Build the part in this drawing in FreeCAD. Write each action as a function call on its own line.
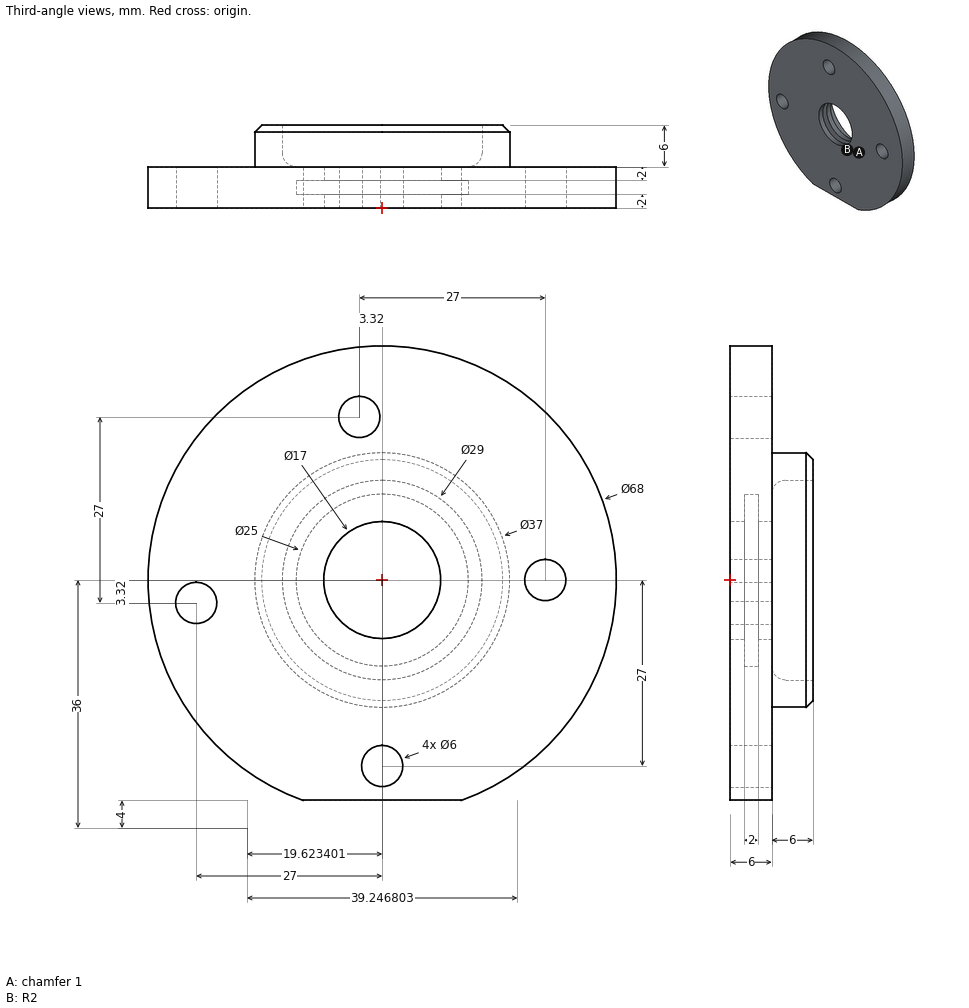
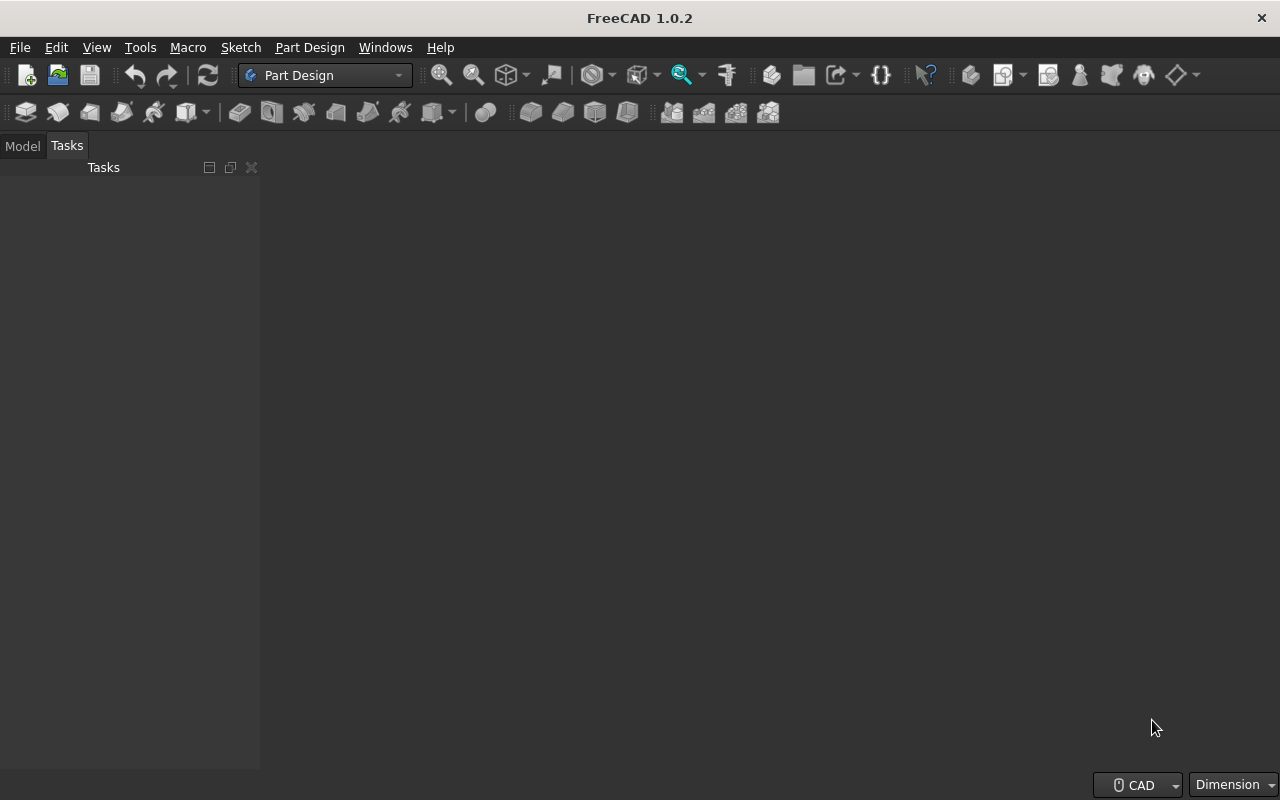
click(26, 76)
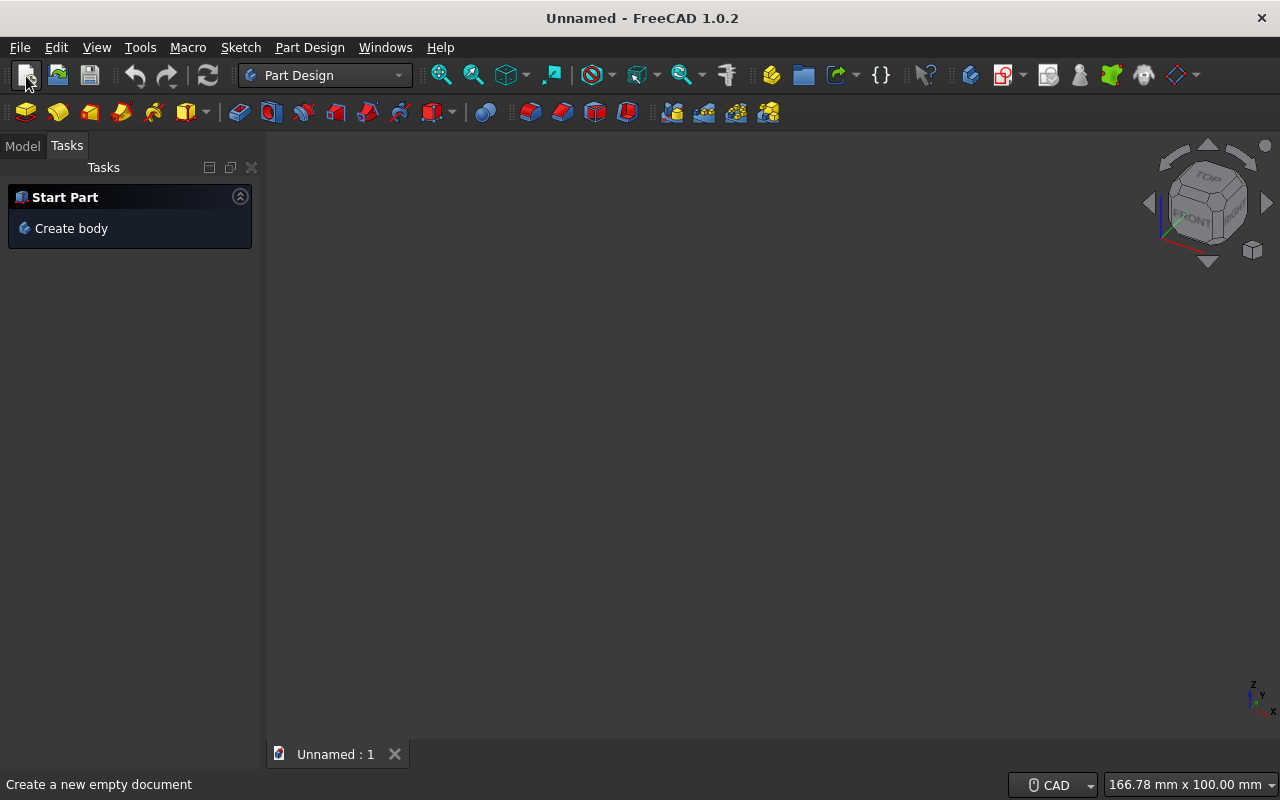
click(1004, 76)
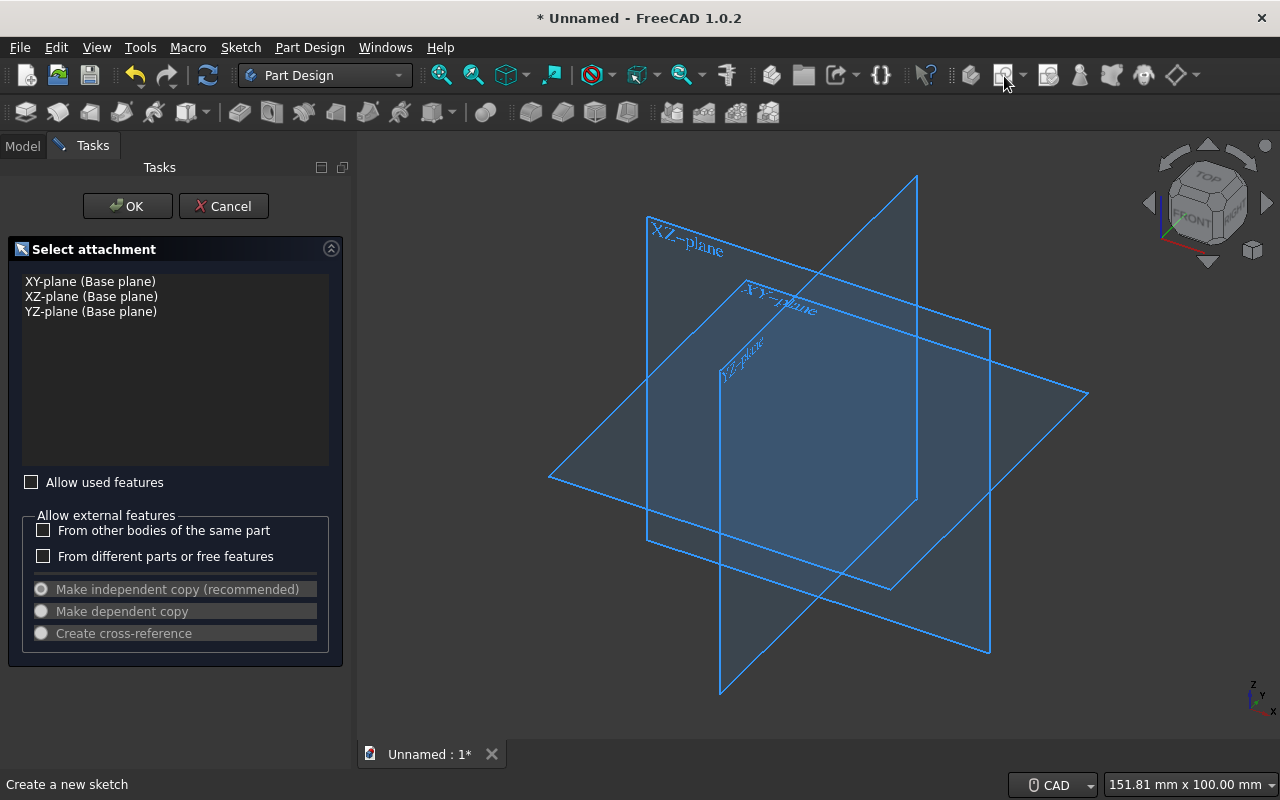
click(82, 296)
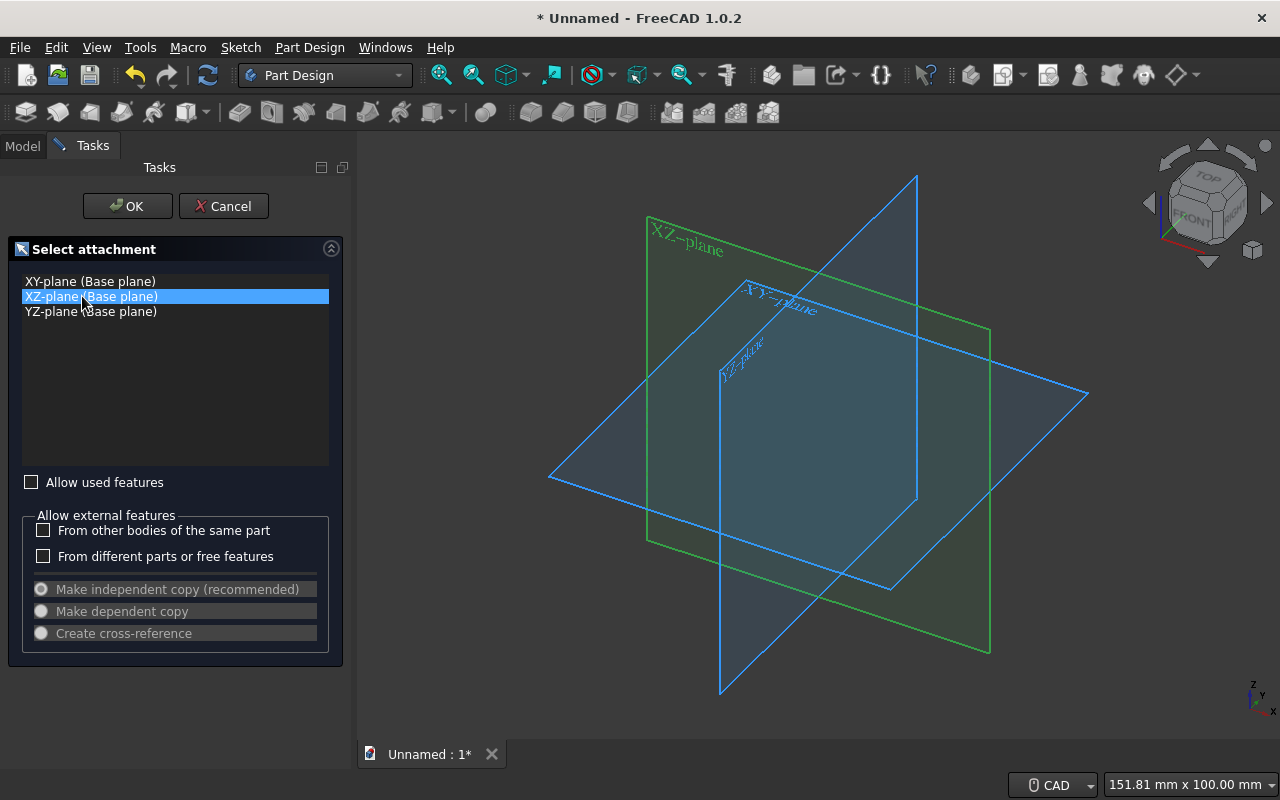
click(128, 206)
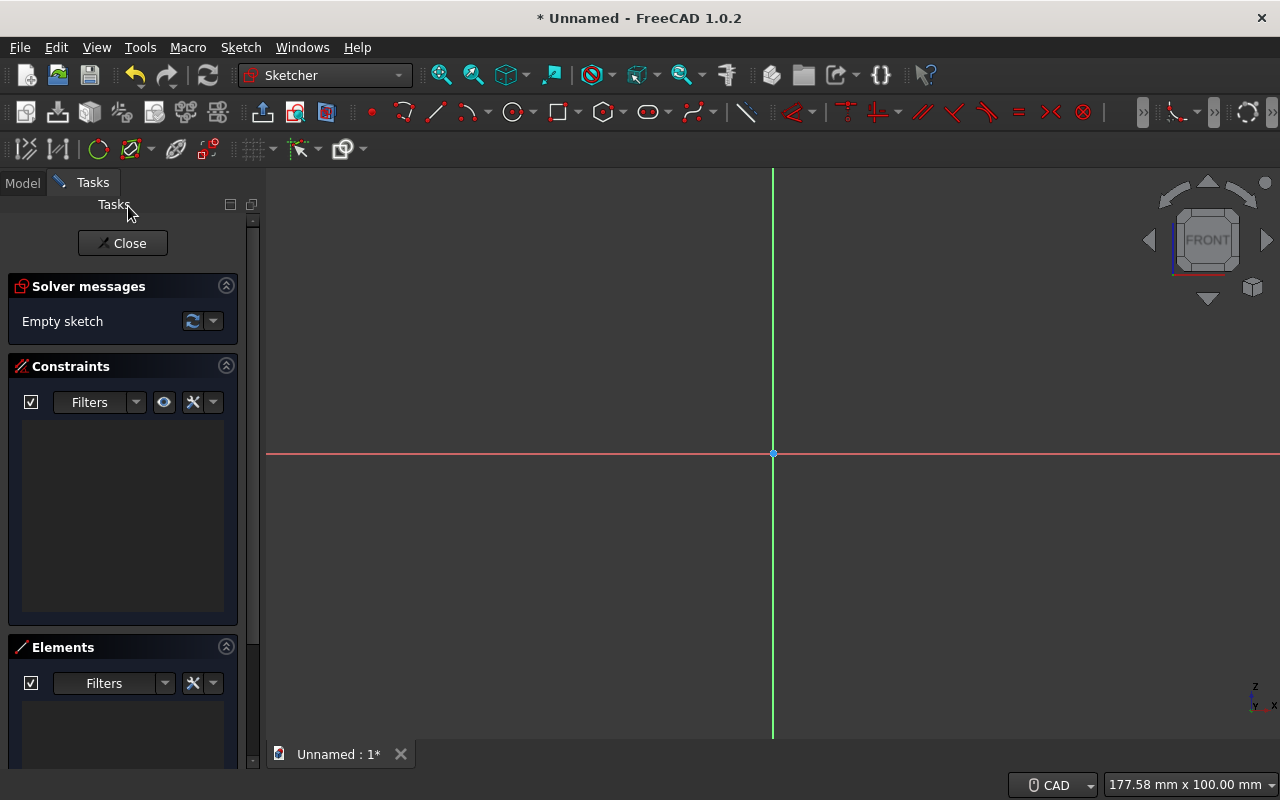
click(514, 112)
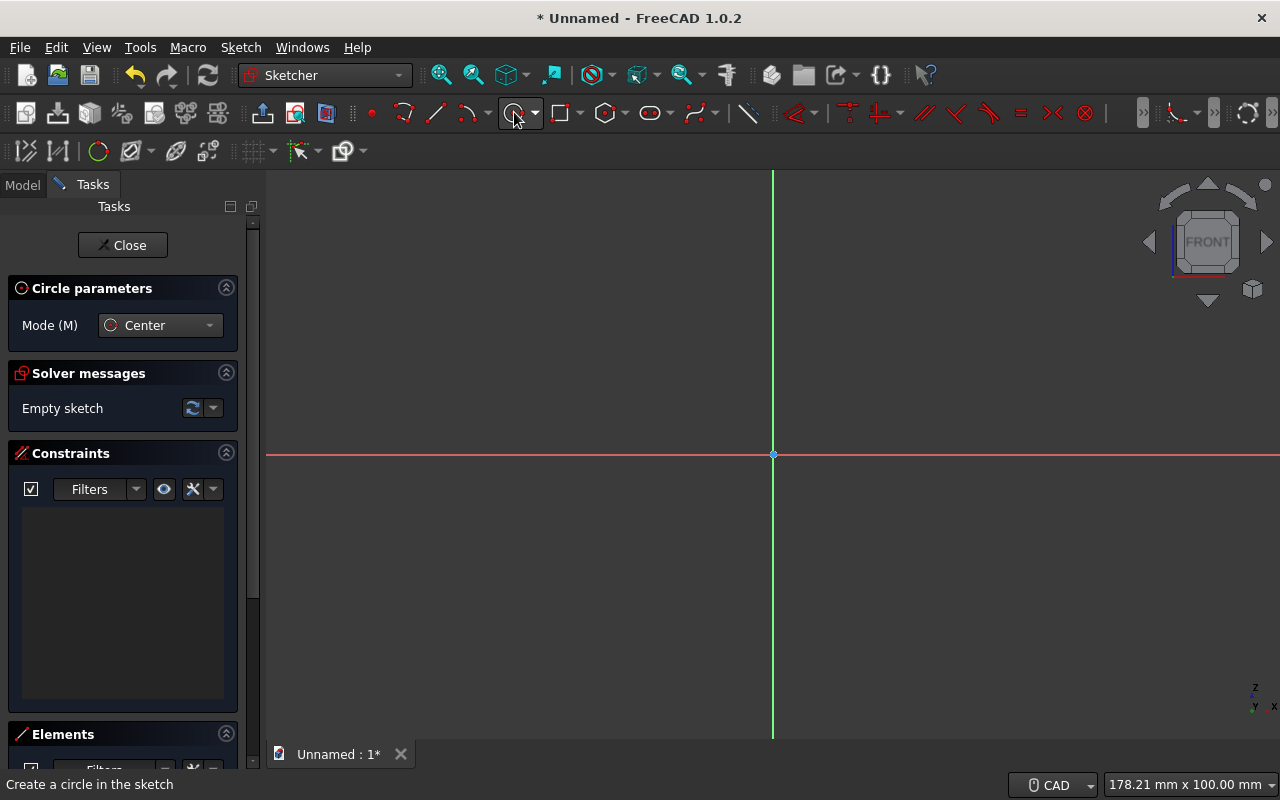
click(773, 454)
click(910, 318)
key(Escape)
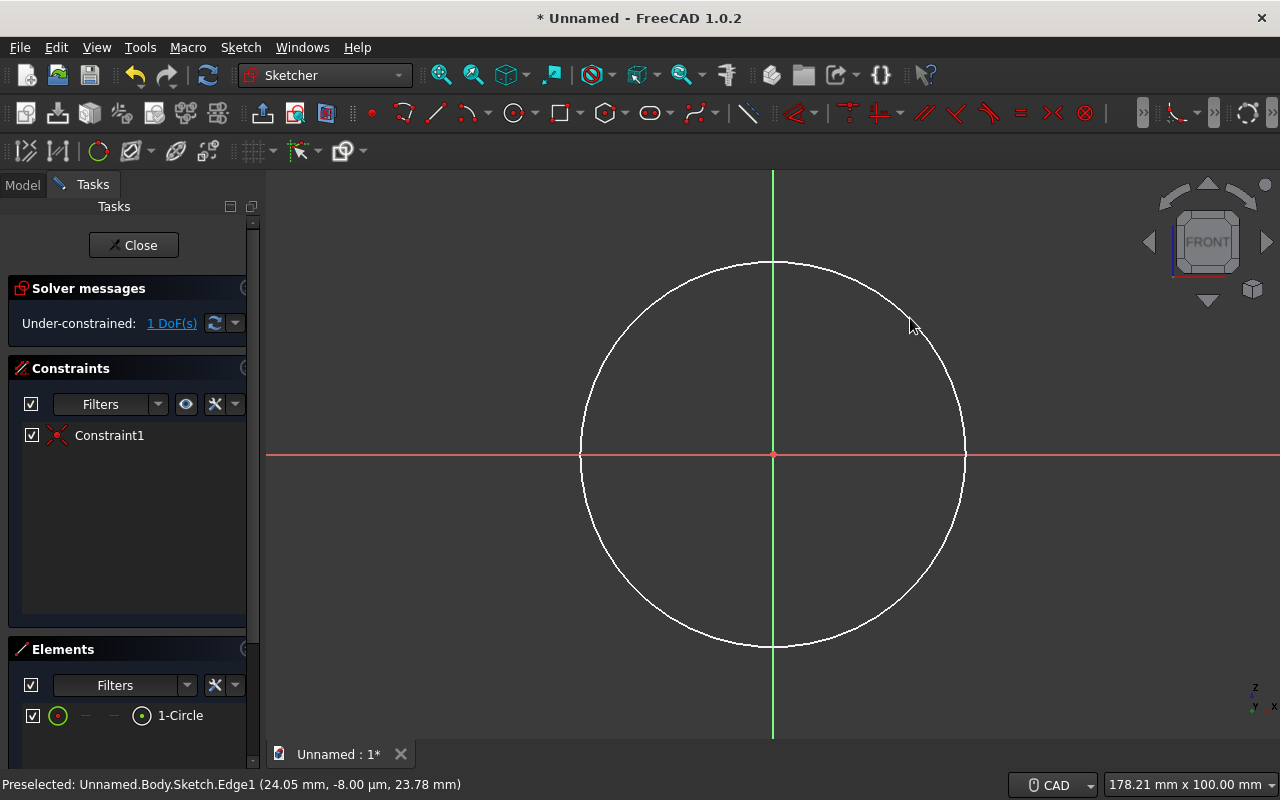
click(794, 114)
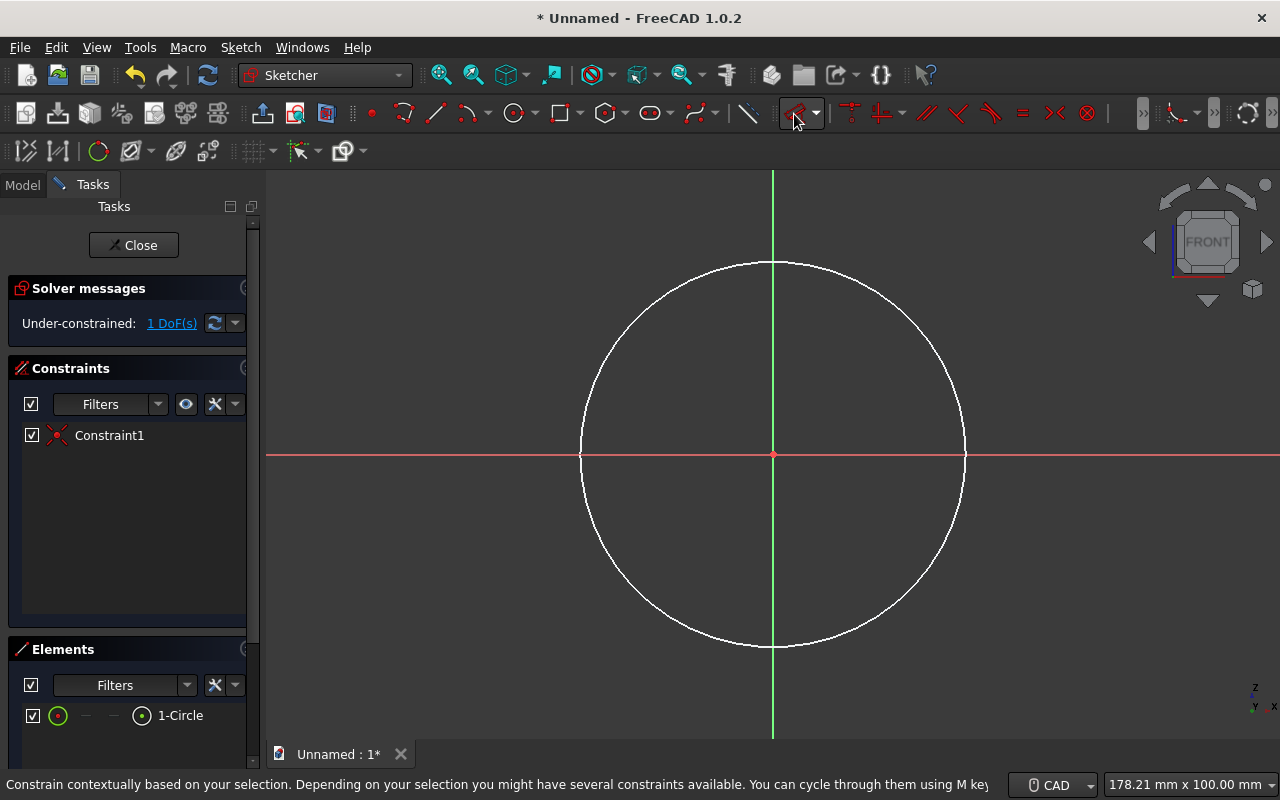
click(909, 318)
click(932, 295)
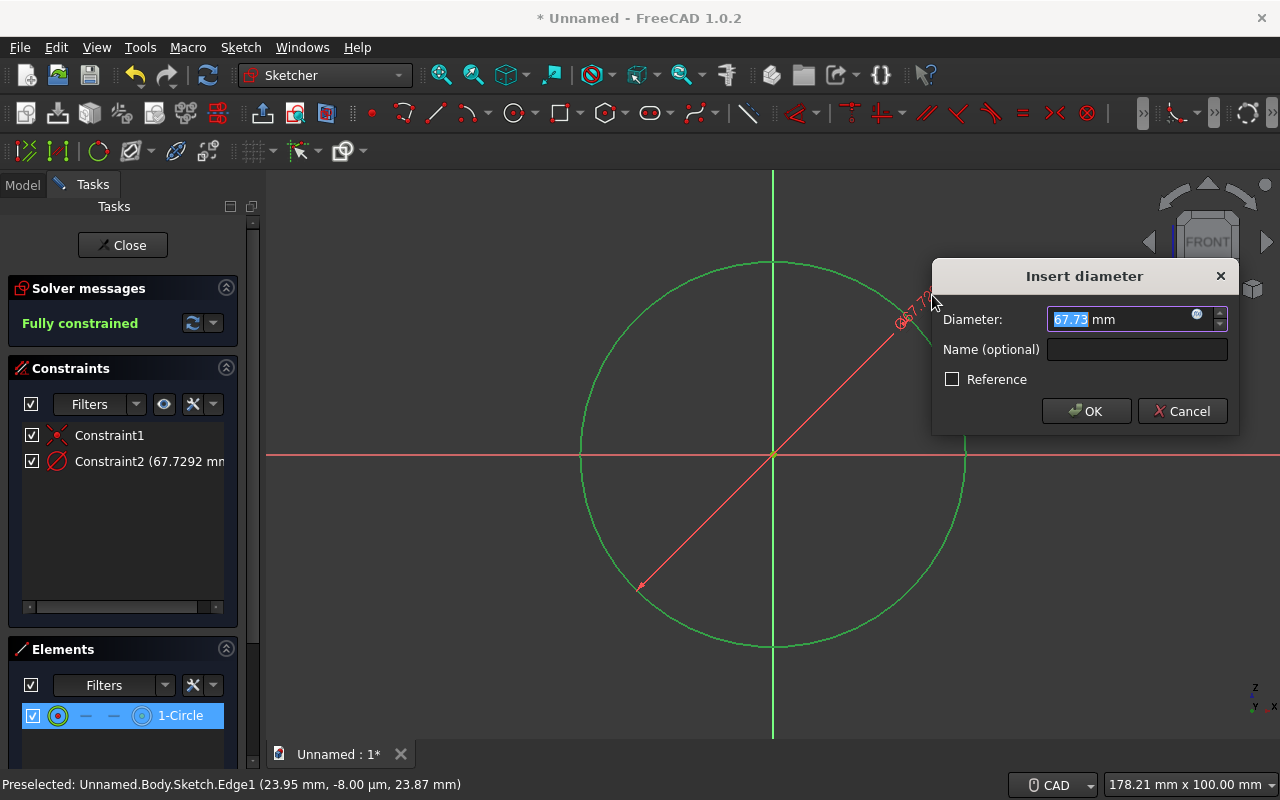
text(68)
key(Return)
key(Escape)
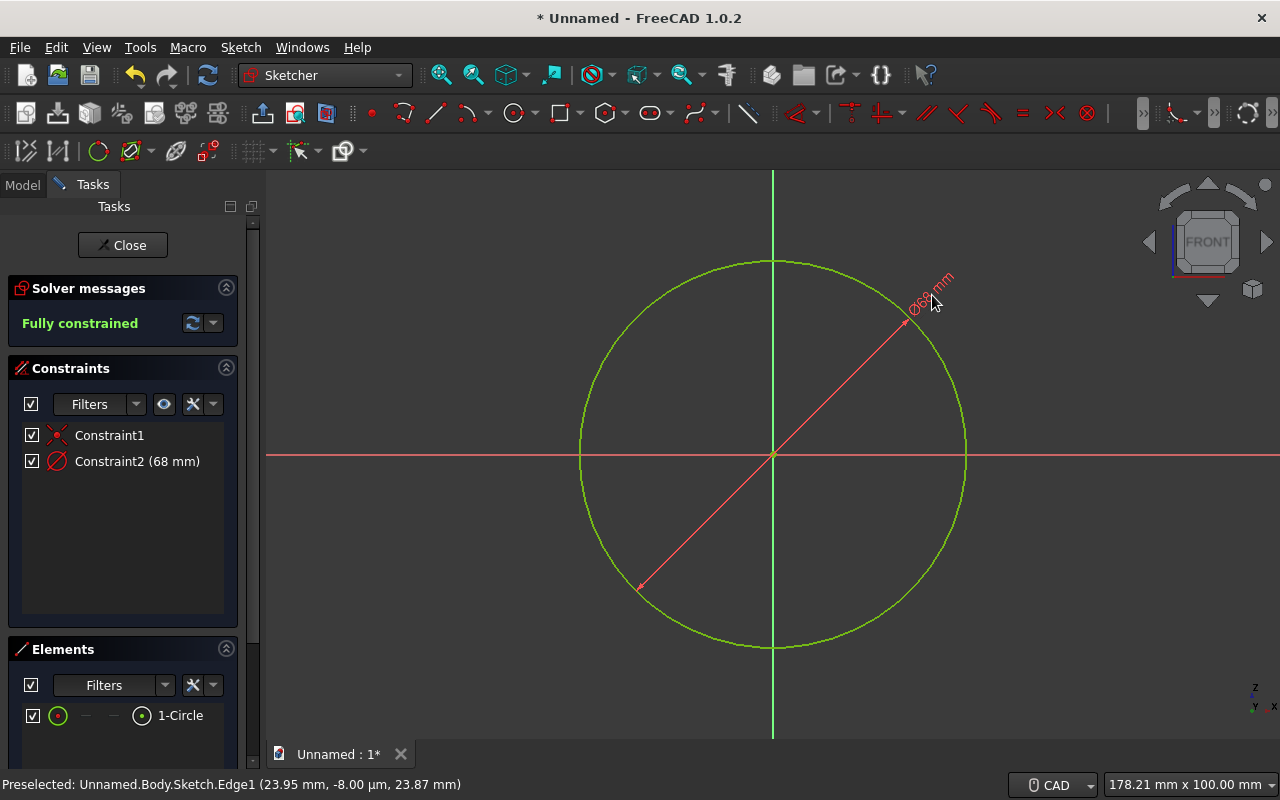
click(123, 245)